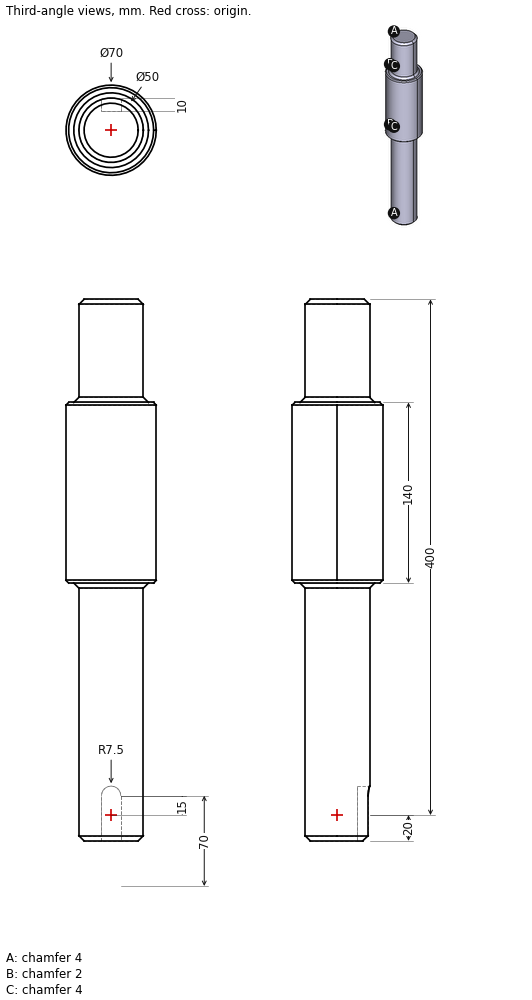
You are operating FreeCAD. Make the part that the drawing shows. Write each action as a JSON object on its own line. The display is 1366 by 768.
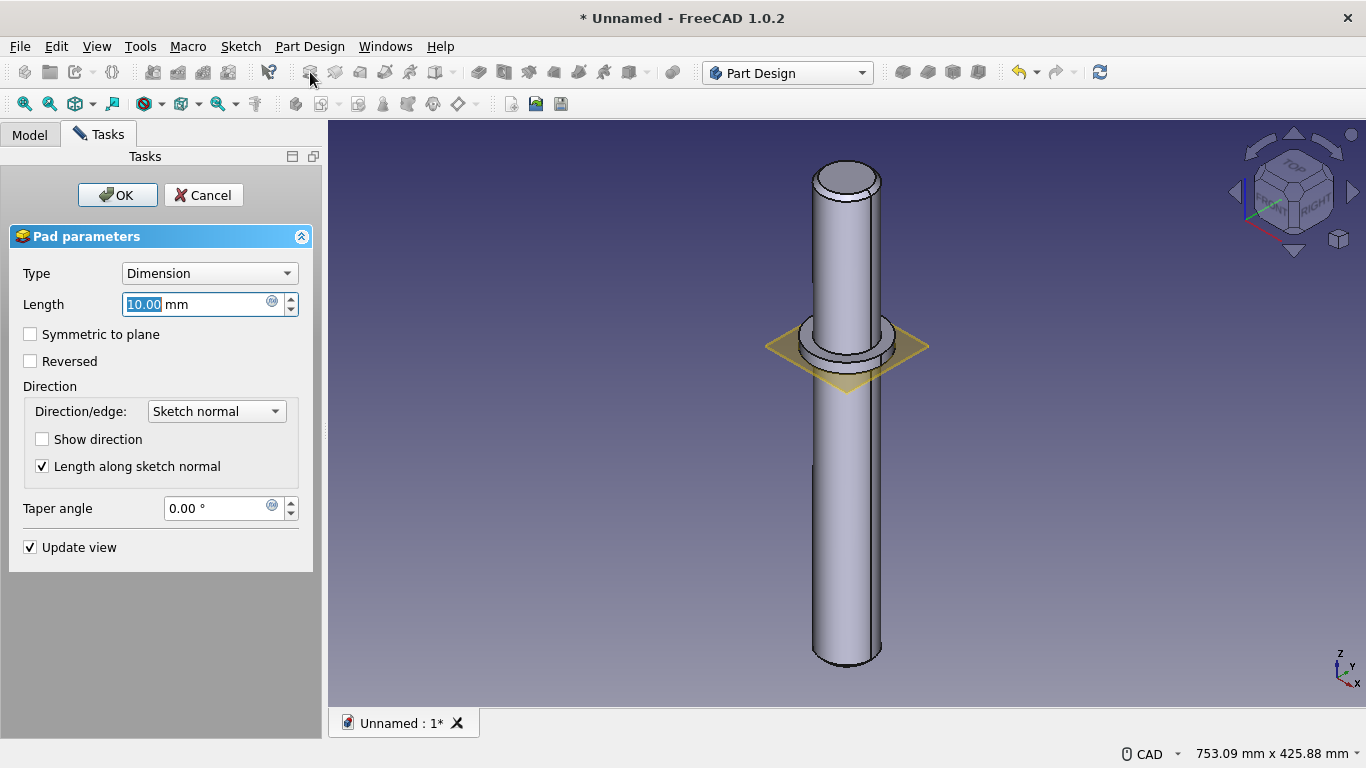
{"action": "type", "text": "140"}
{"action": "key", "text": "Tab"}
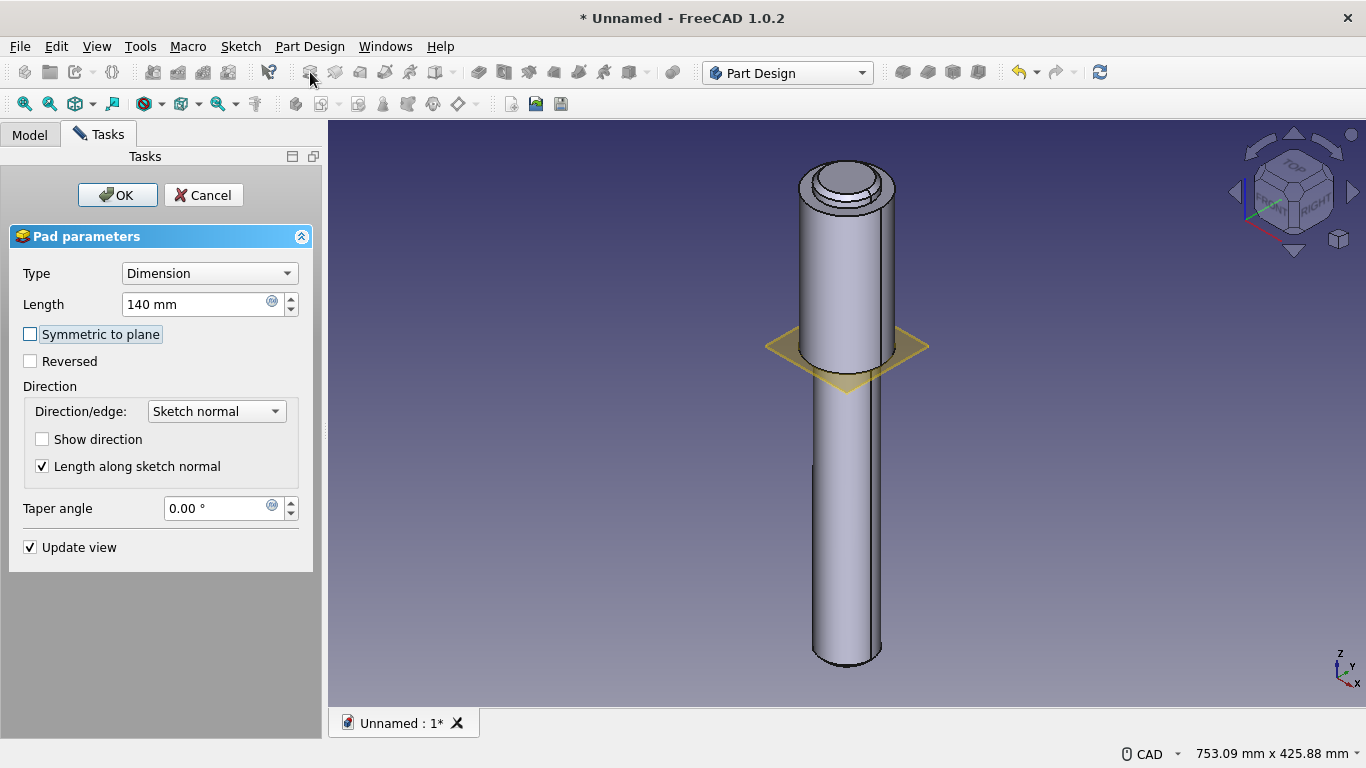
{"action": "left_click", "coordinate": [31, 334]}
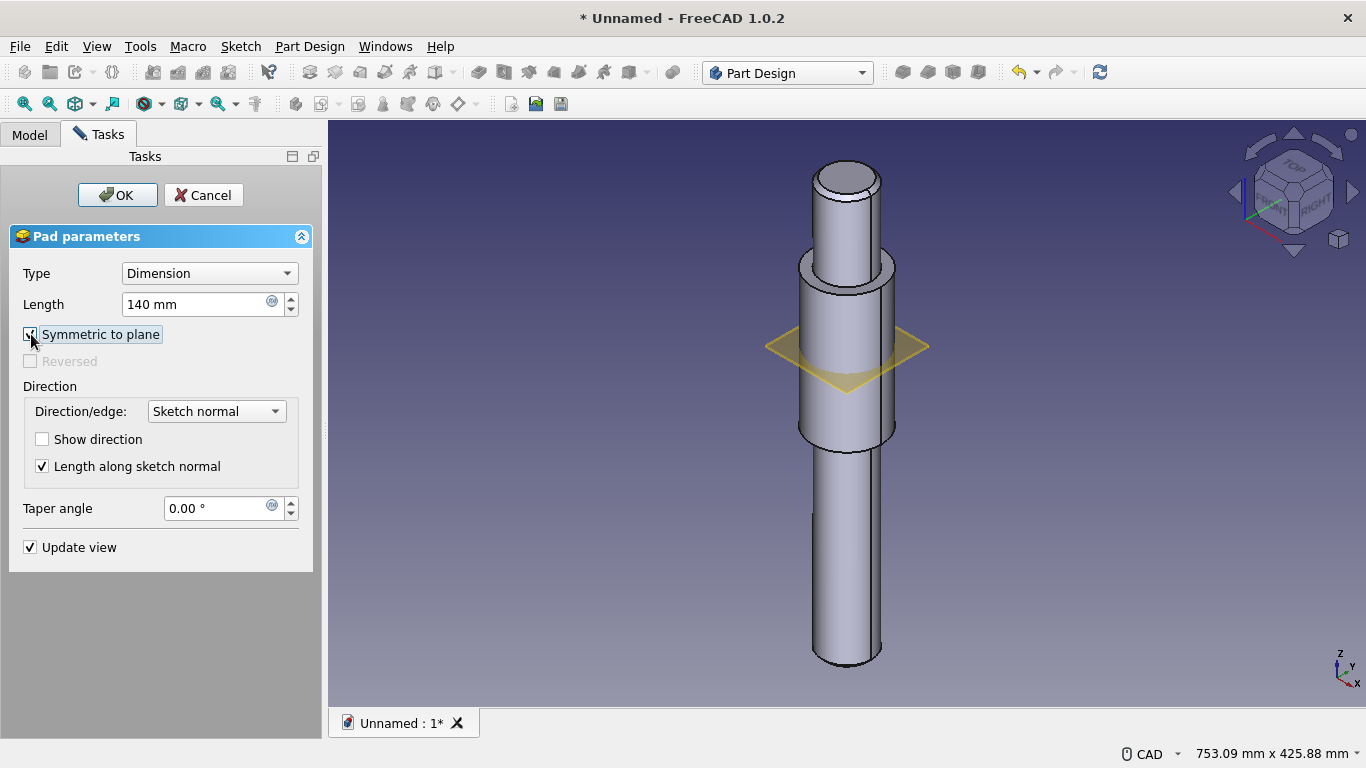
{"action": "left_click", "coordinate": [118, 195]}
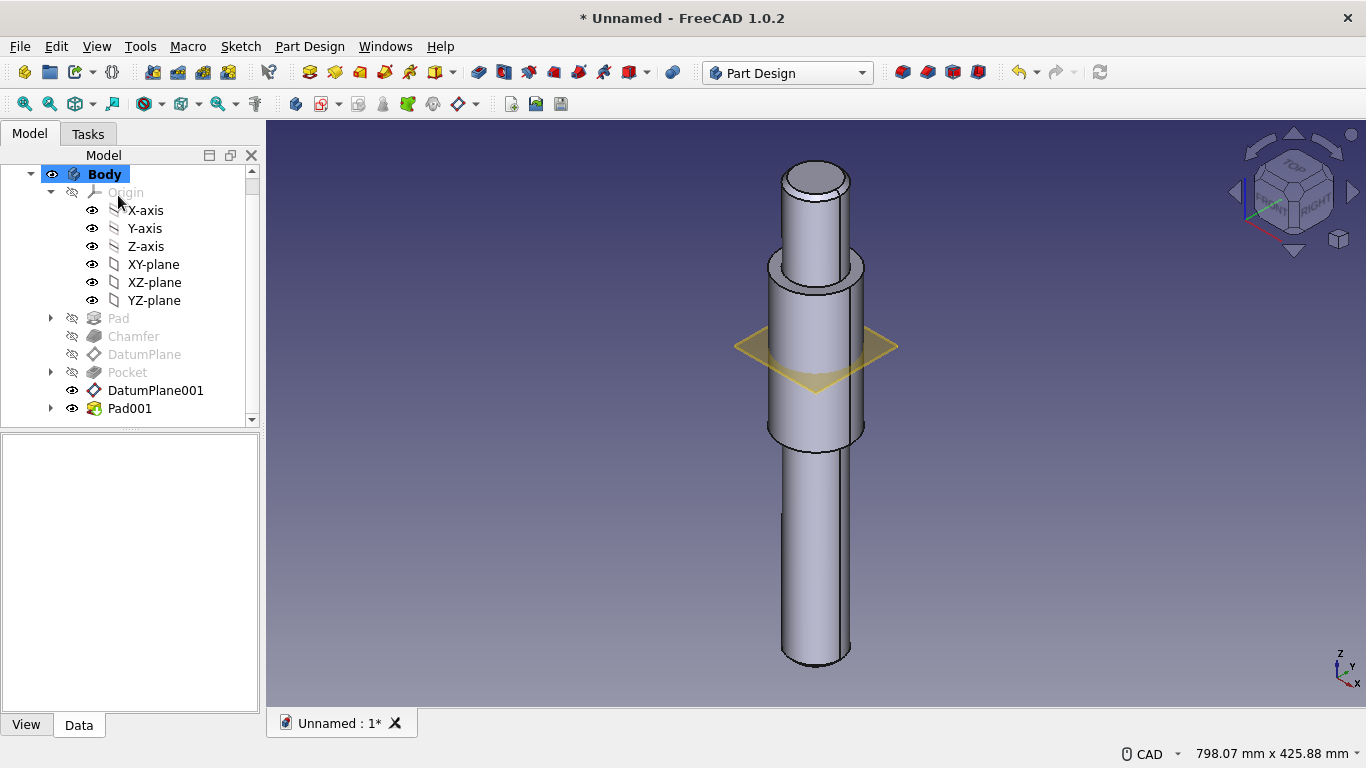
{"action": "left_click", "coordinate": [117, 390]}
{"action": "key", "text": "space"}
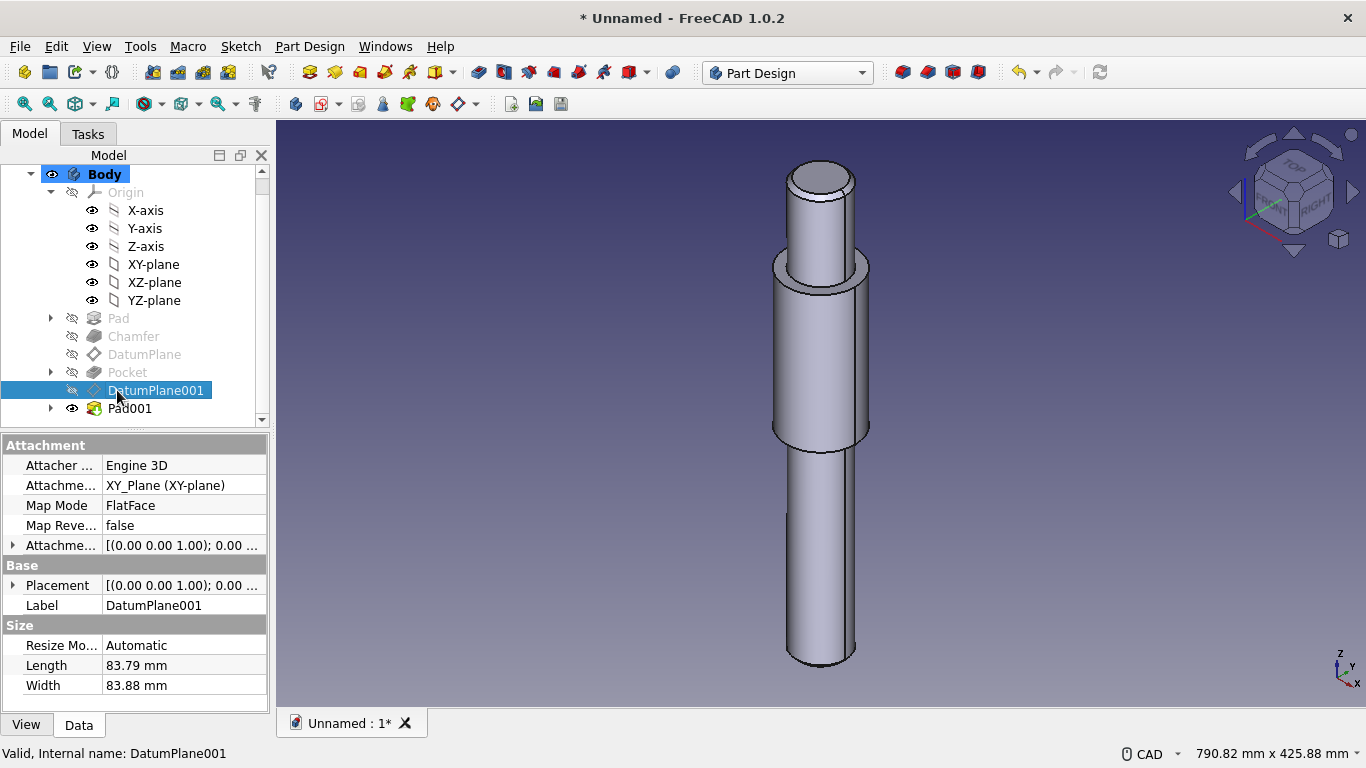
{"action": "left_click", "coordinate": [778, 279]}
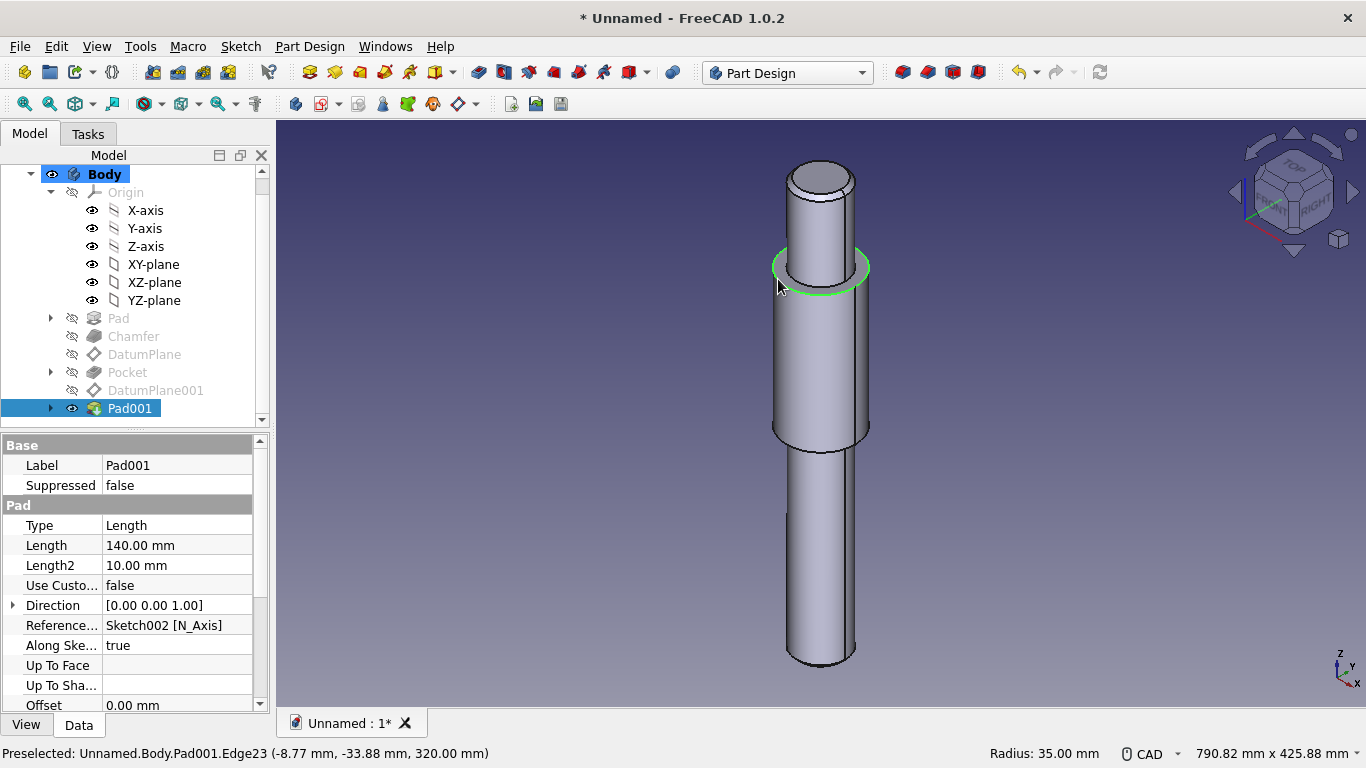
{"action": "key", "text": "2"}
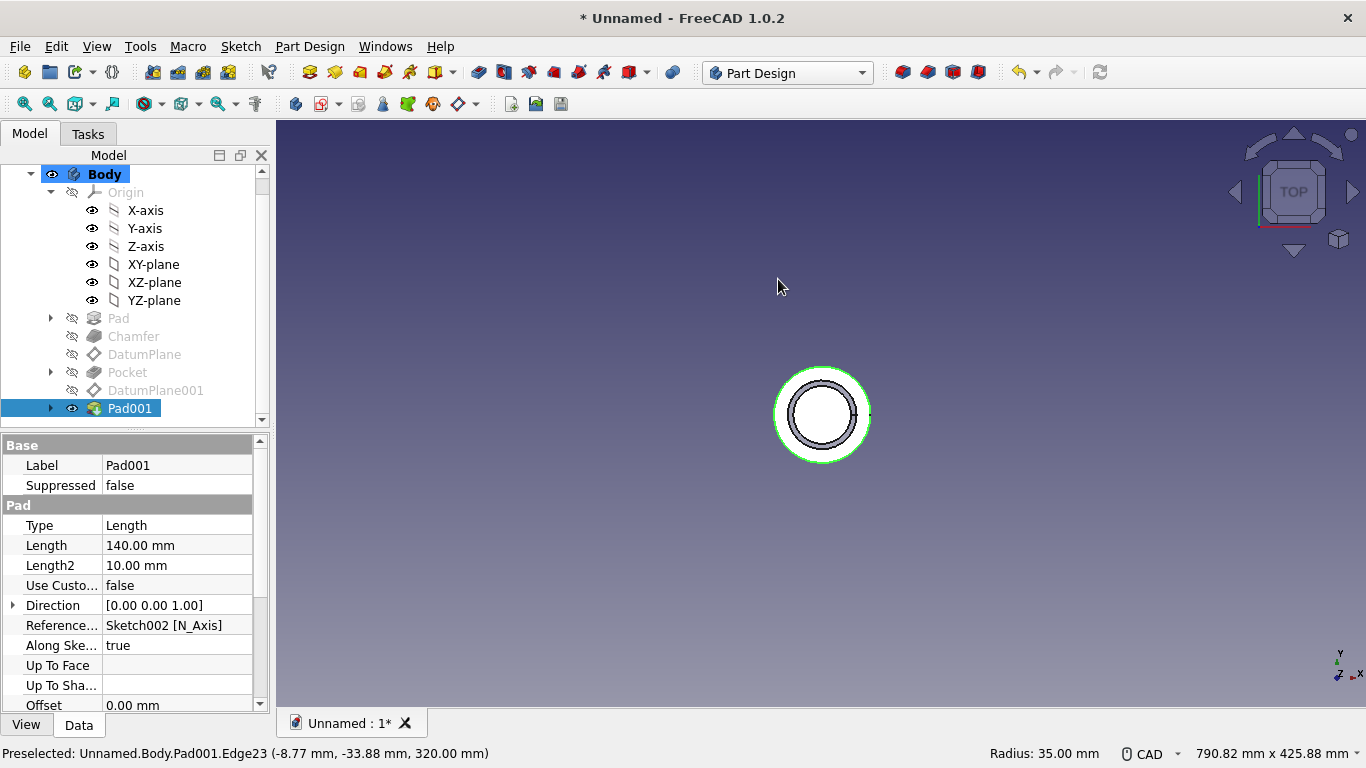
{"action": "left_click", "coordinate": [25, 104]}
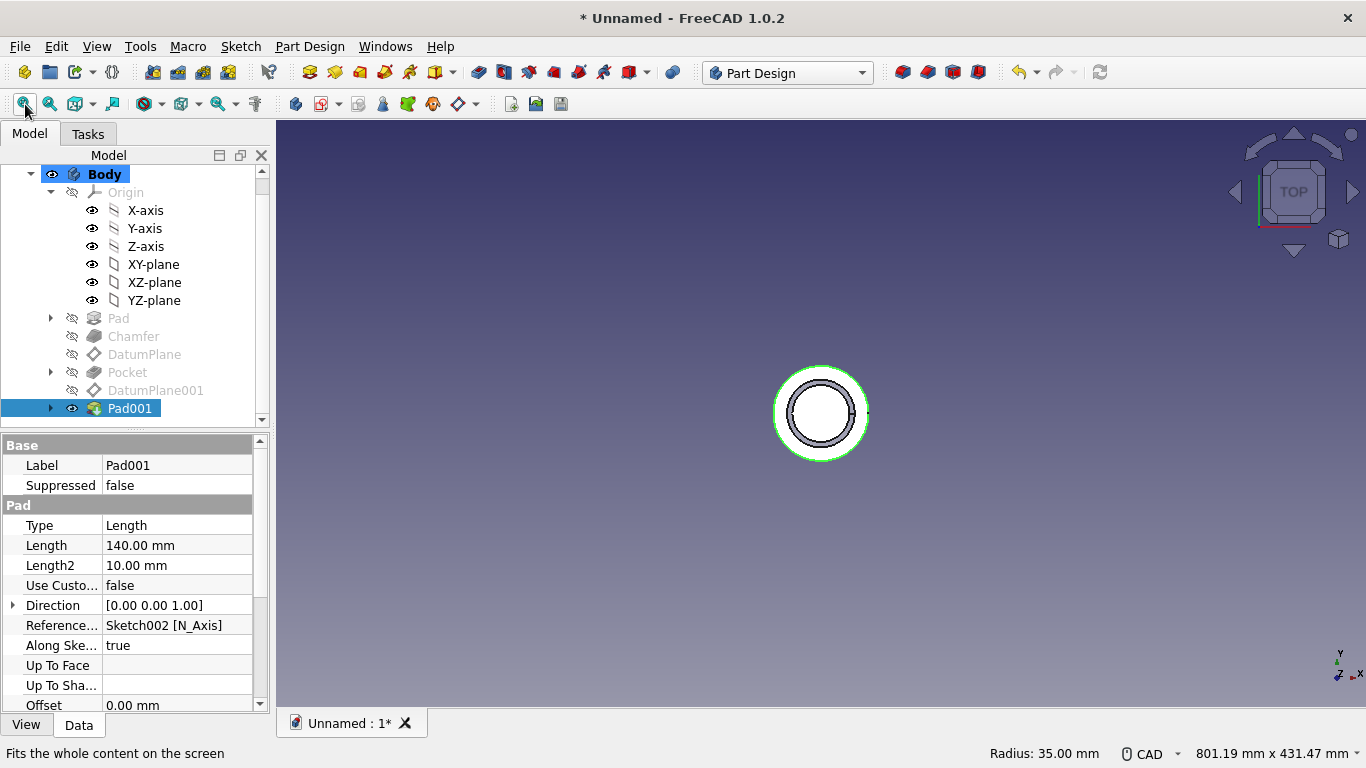
{"action": "key", "text": "0"}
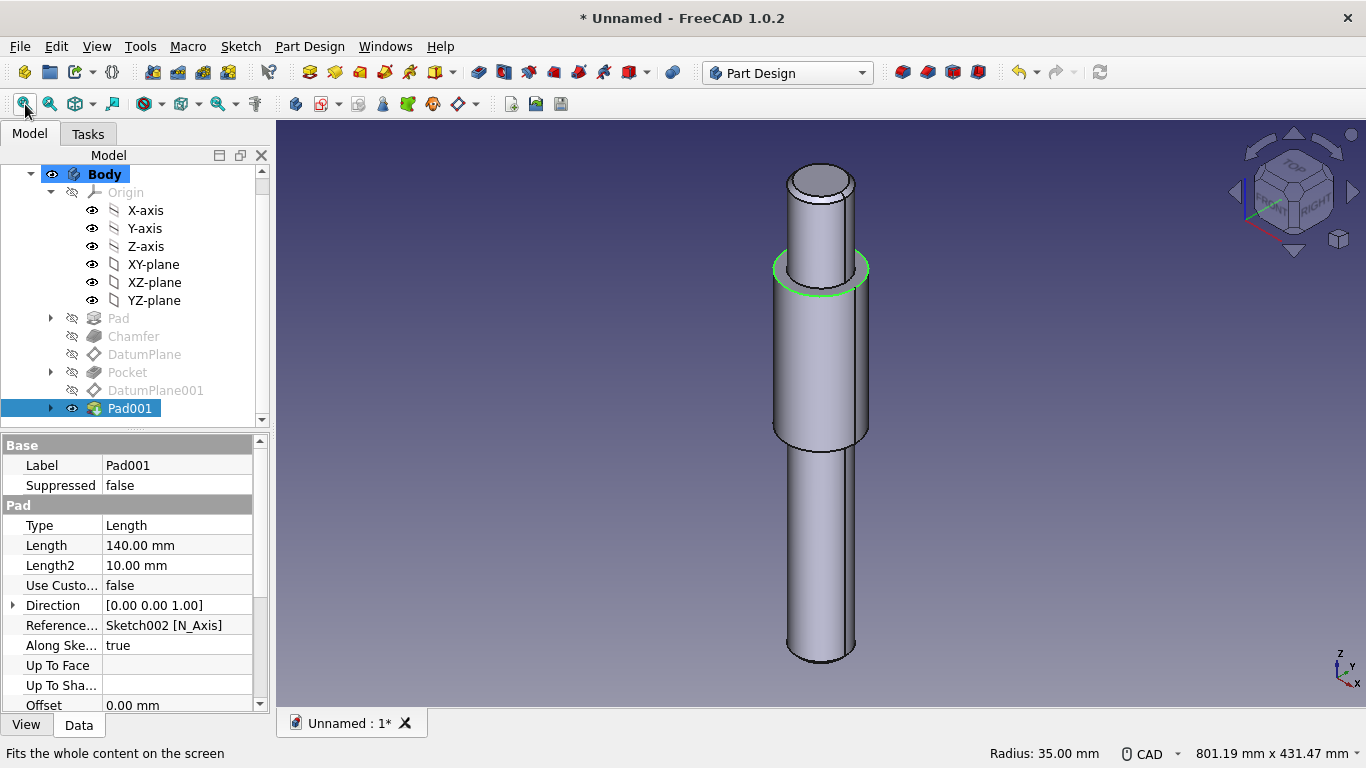
{"action": "left_click", "coordinate": [778, 436], "text": "ctrl"}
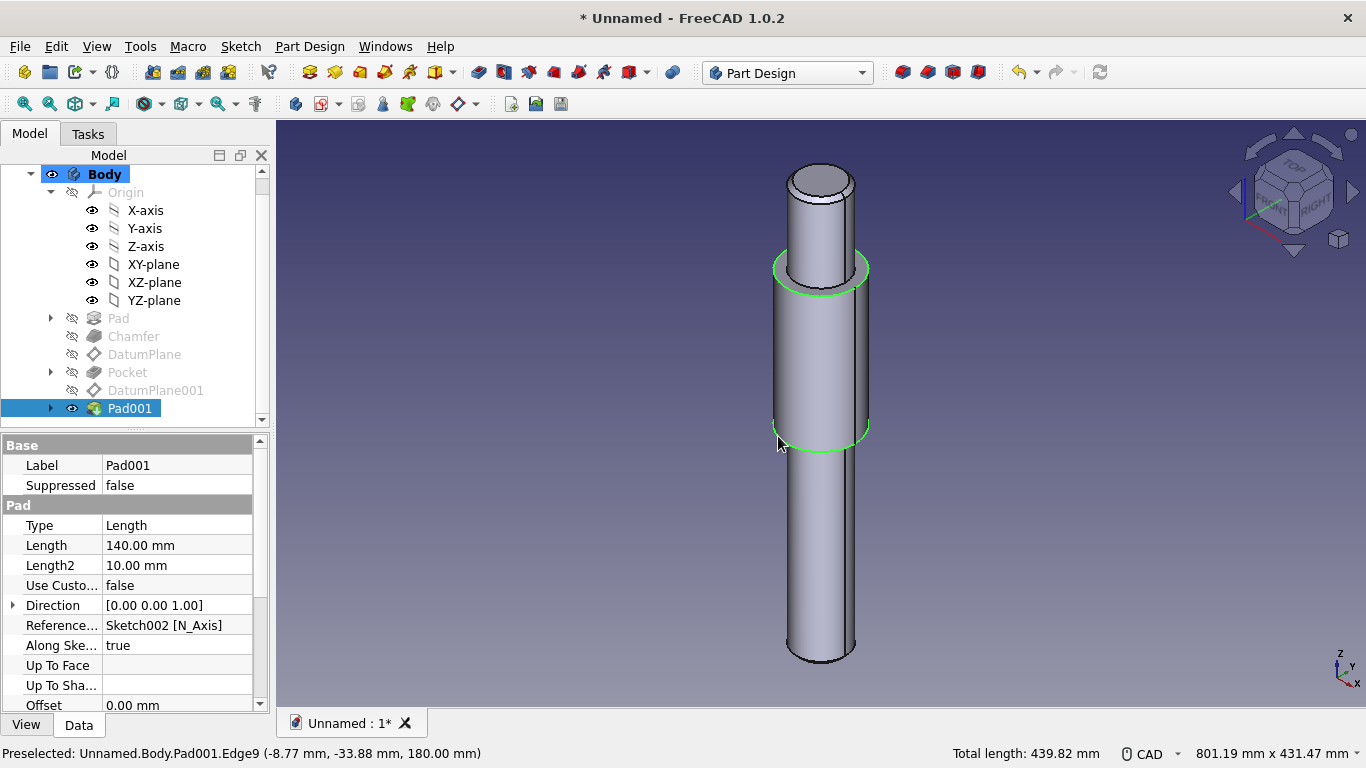
{"action": "left_click", "coordinate": [928, 72]}